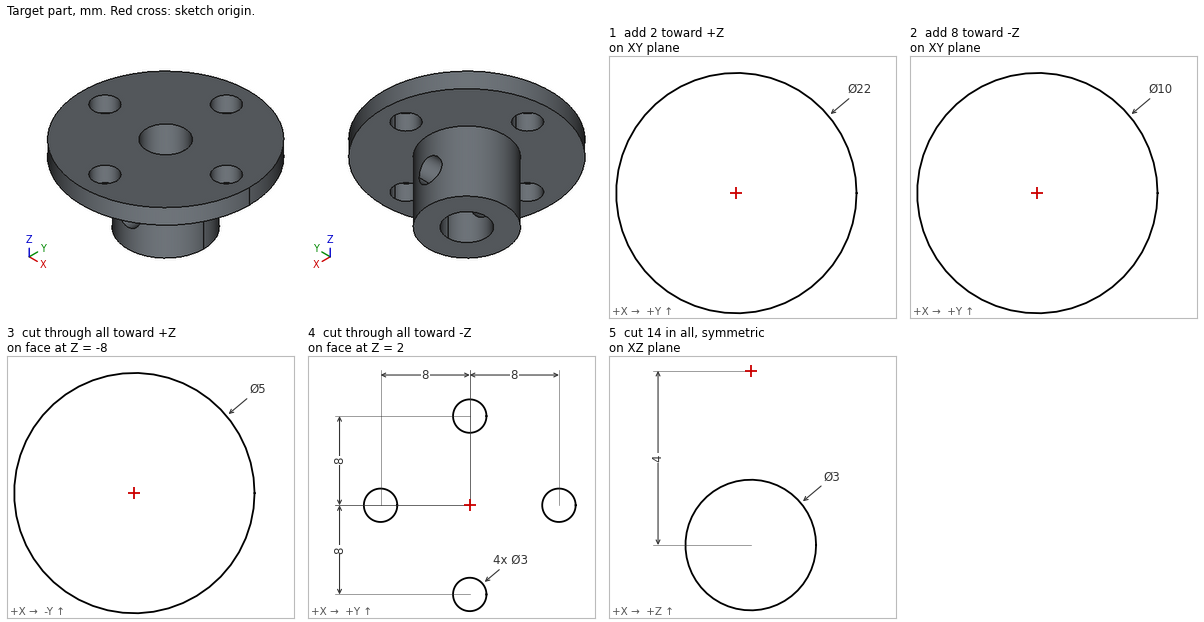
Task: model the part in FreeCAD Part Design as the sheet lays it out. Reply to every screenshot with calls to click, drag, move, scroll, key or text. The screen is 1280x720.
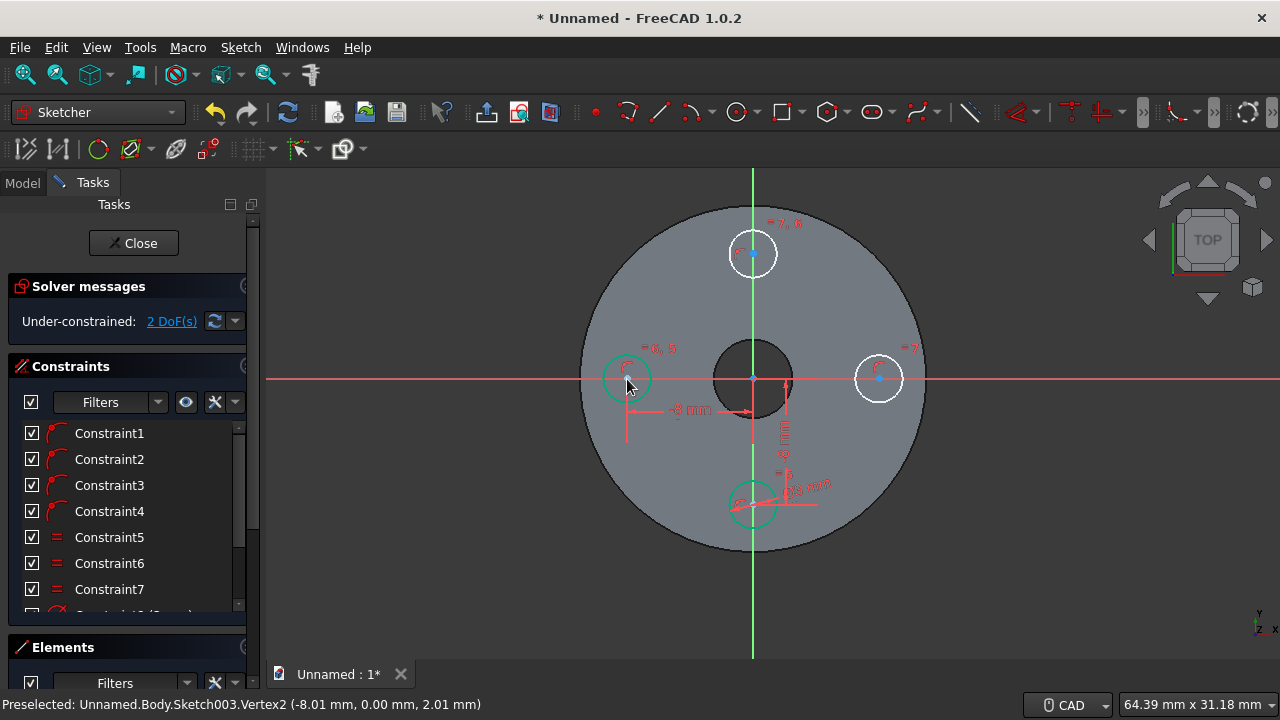
click(753, 254)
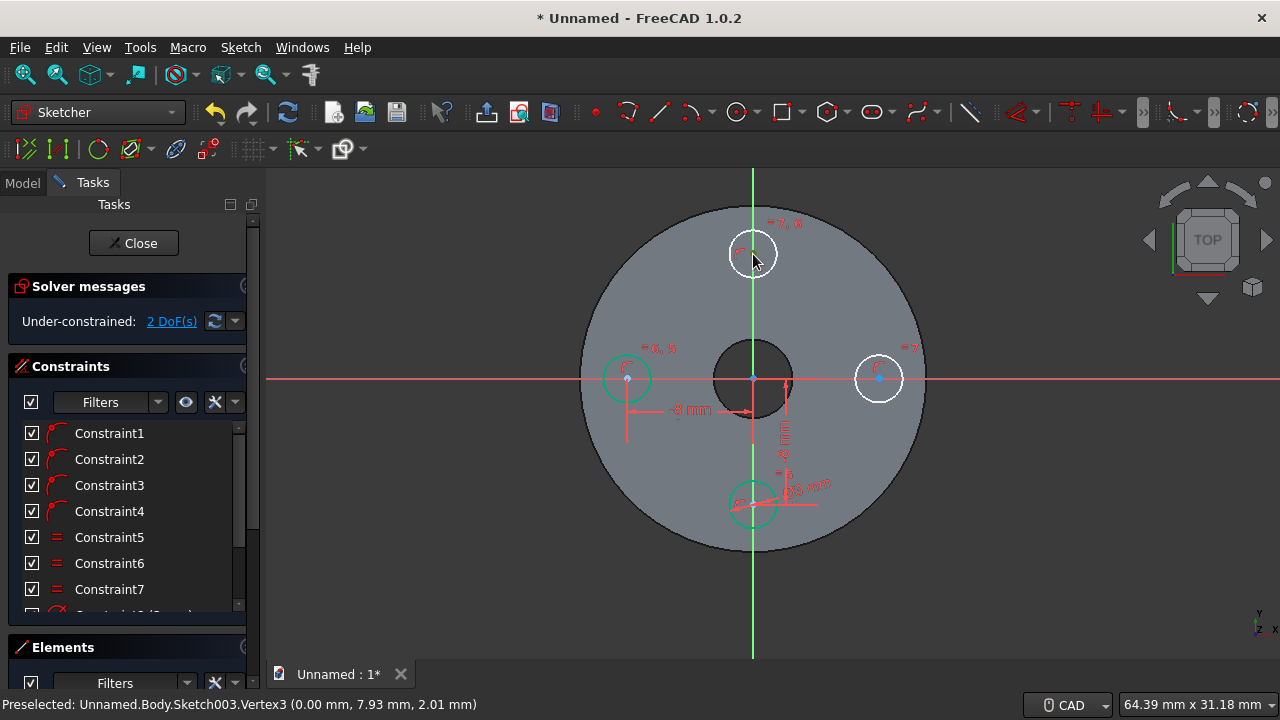
key(i)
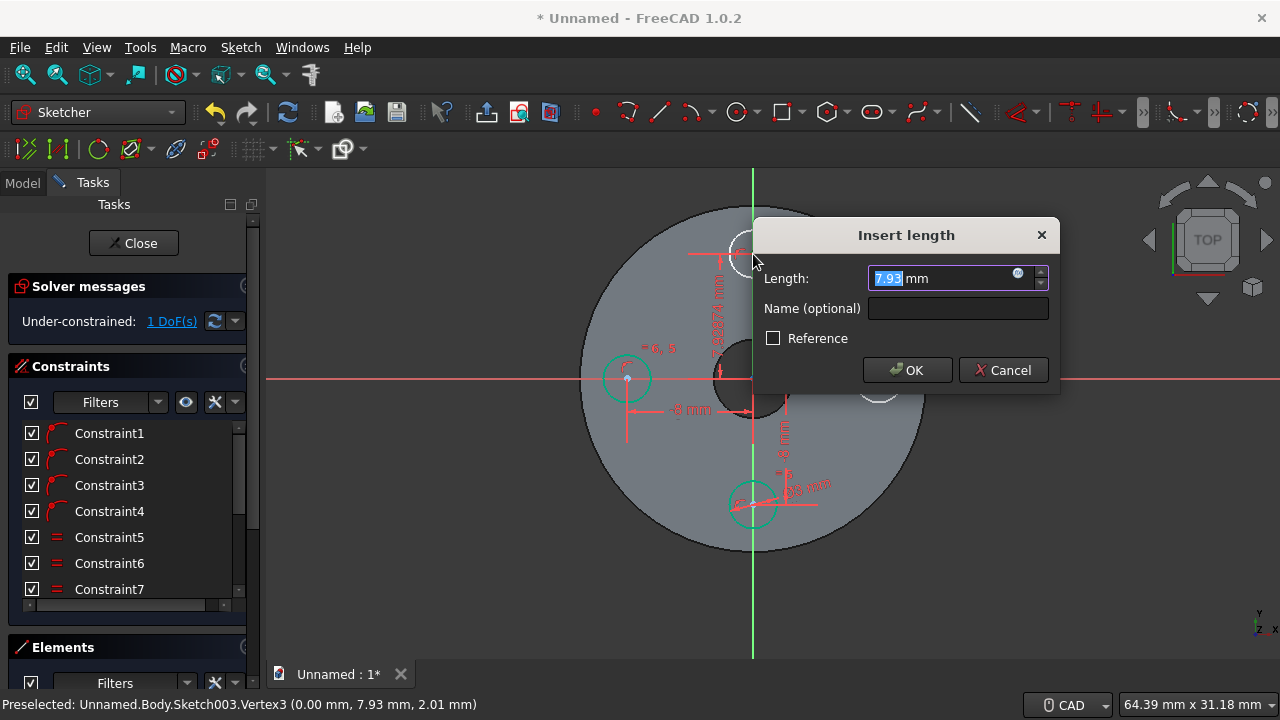
text(8)
key(Return)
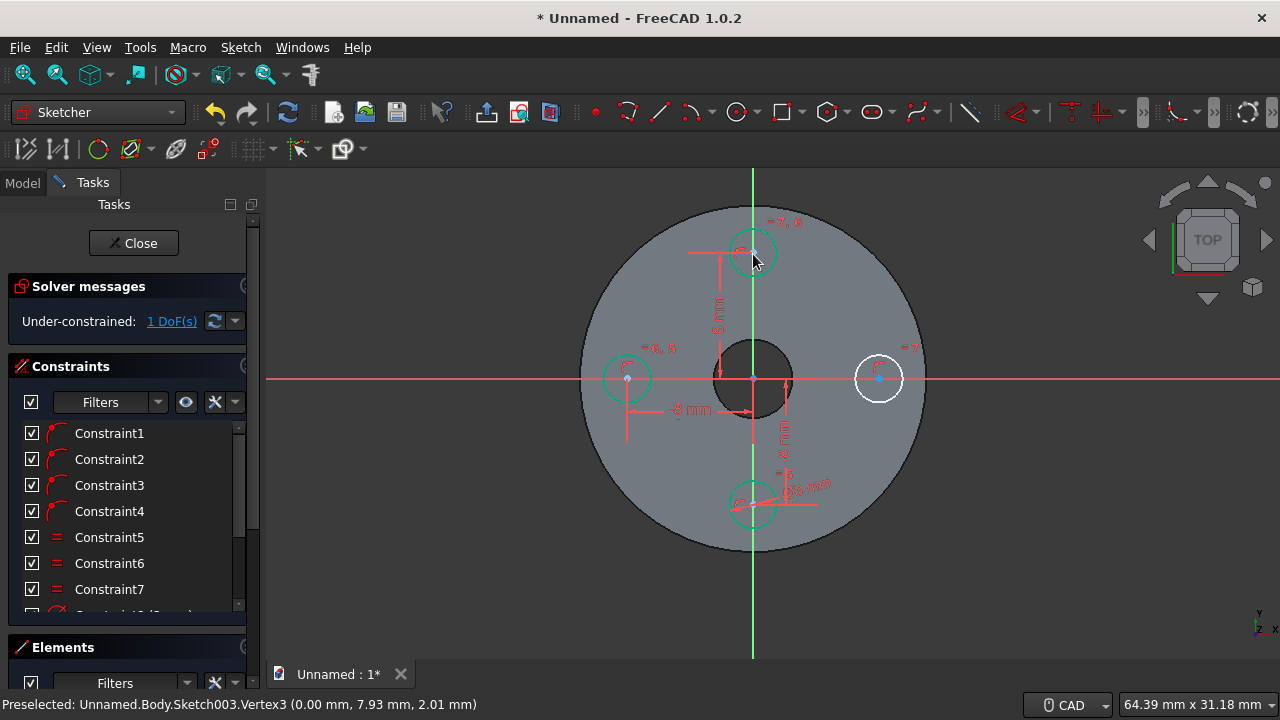
click(879, 379)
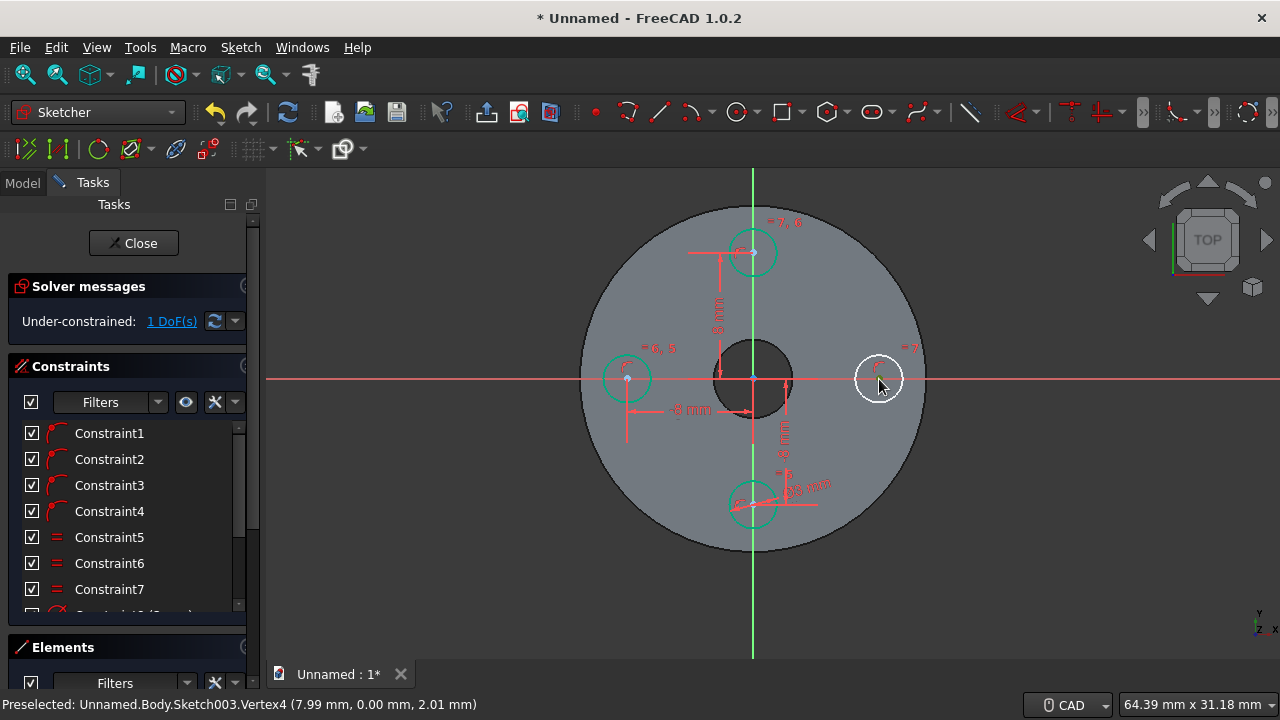
key(l)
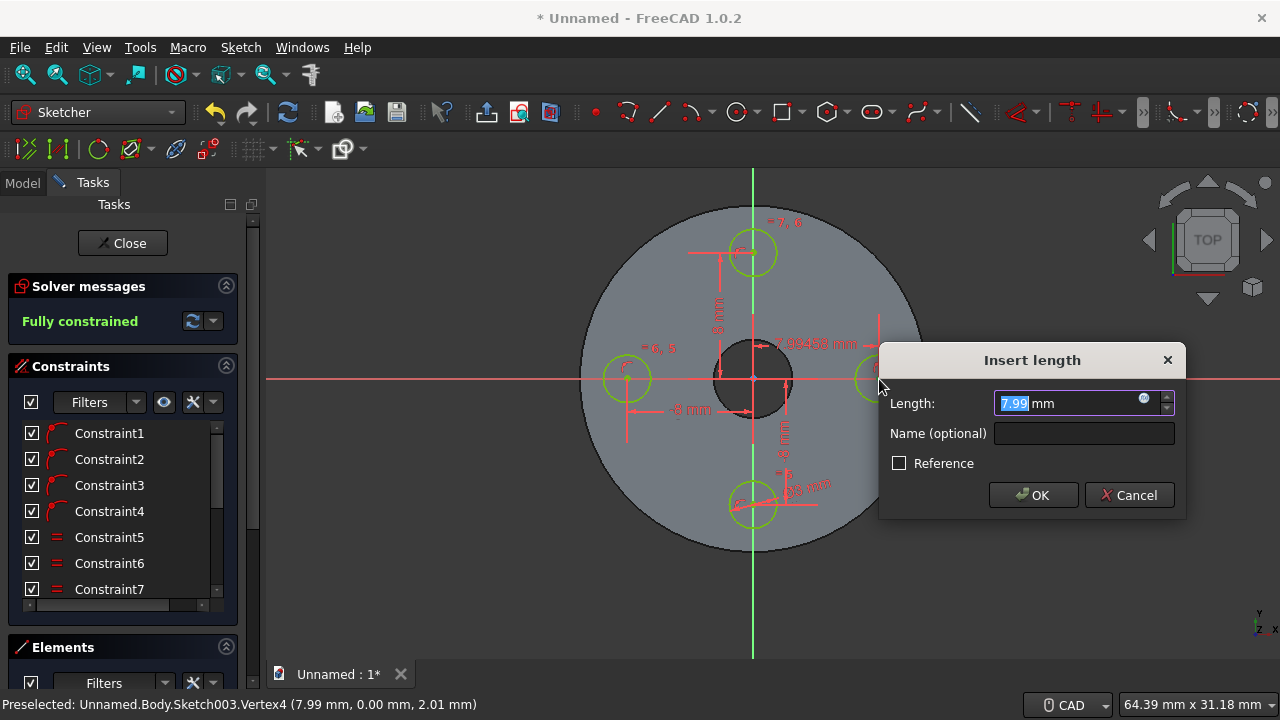
text(8)
key(Return)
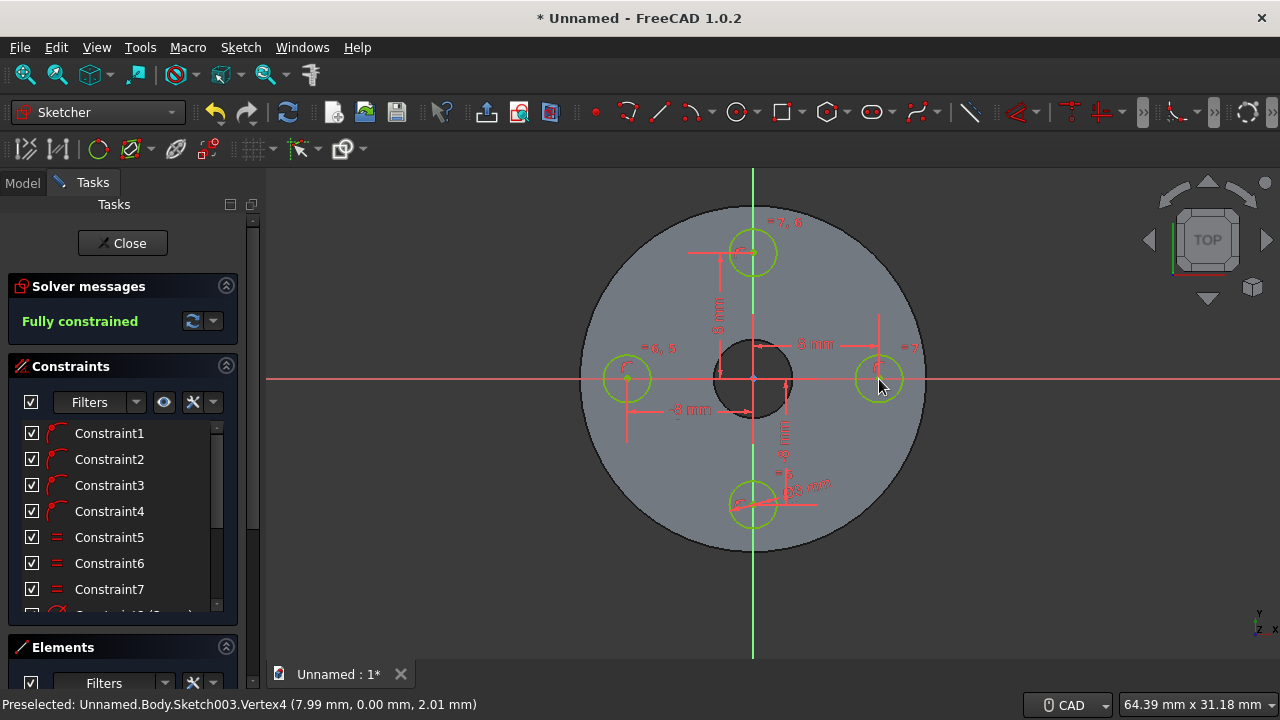
click(123, 243)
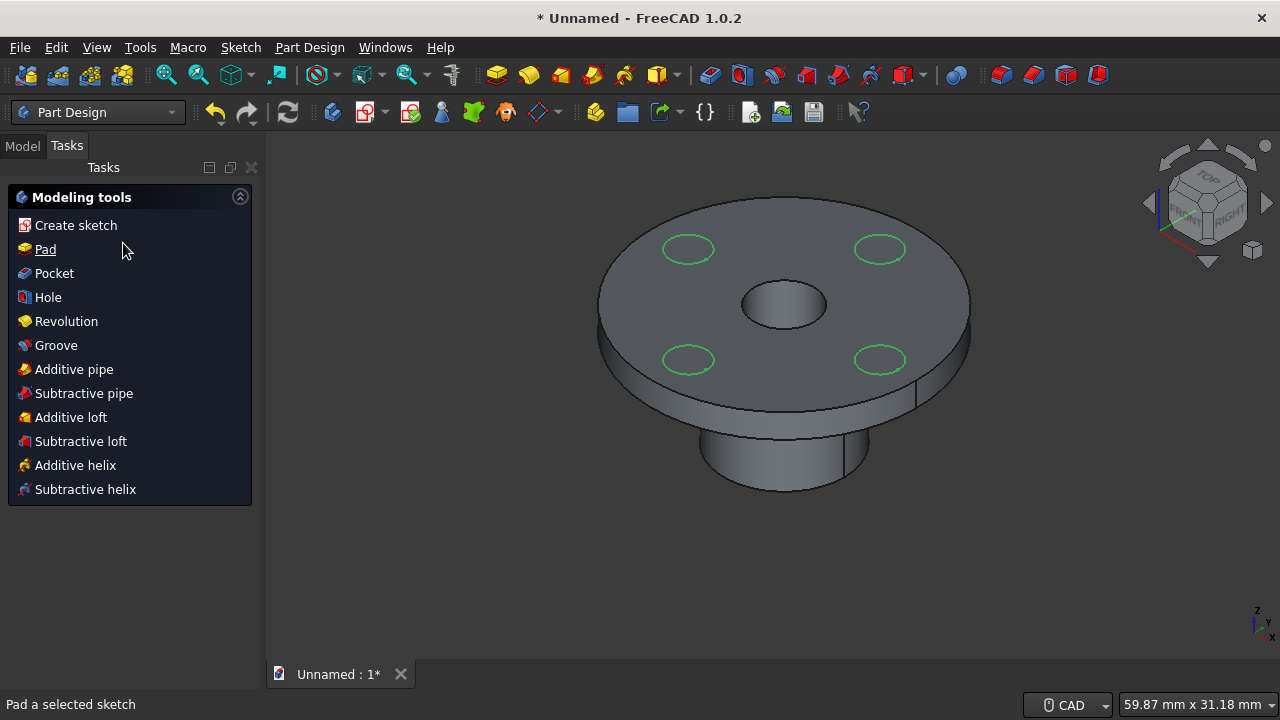
click(712, 76)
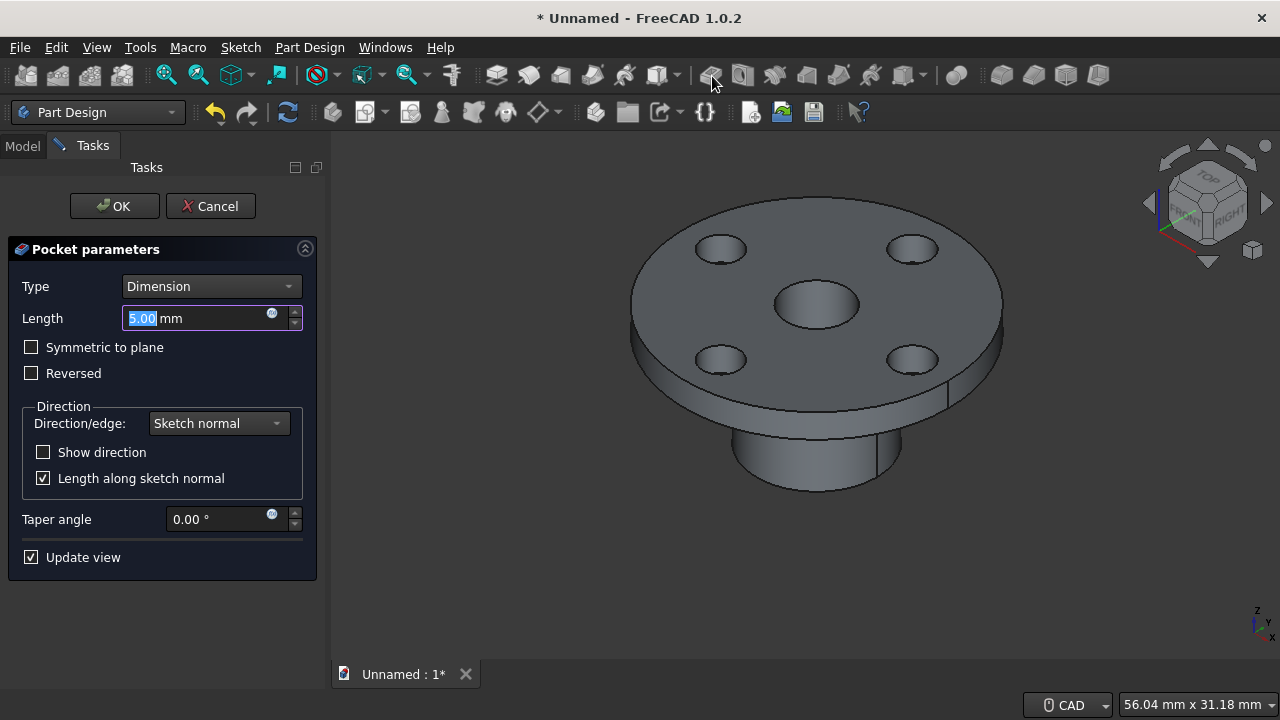
click(212, 286)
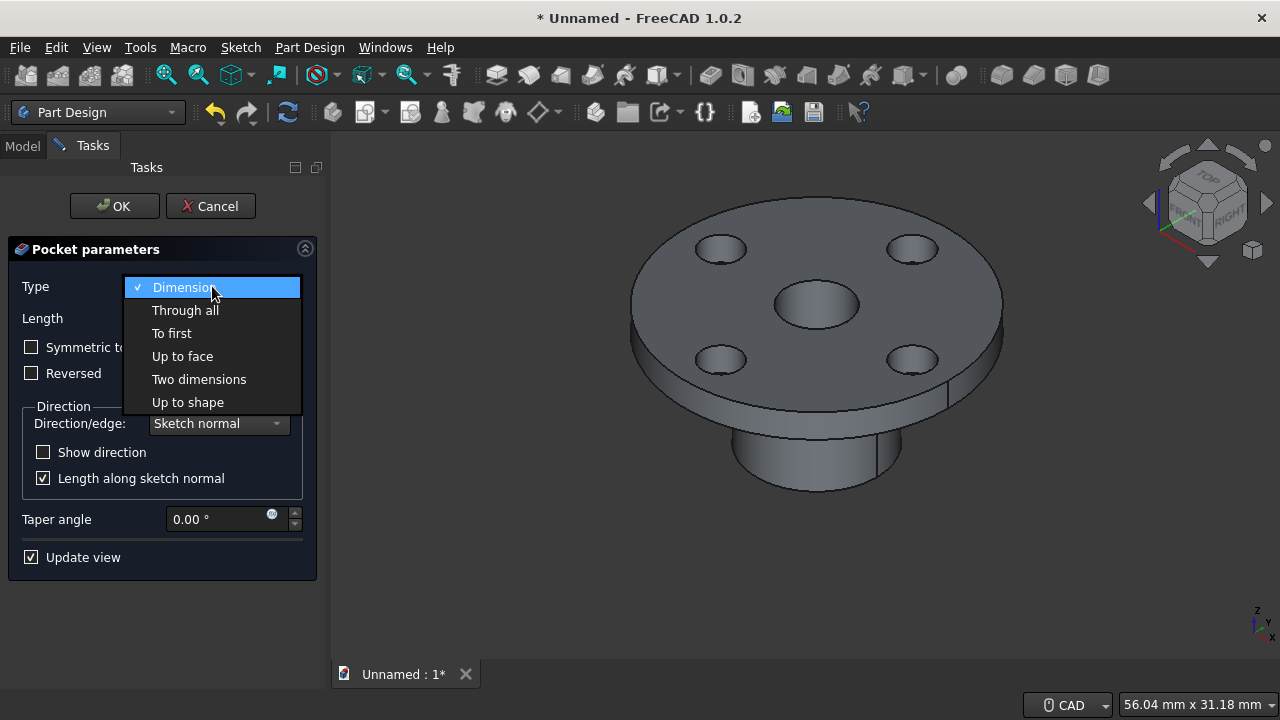
click(212, 310)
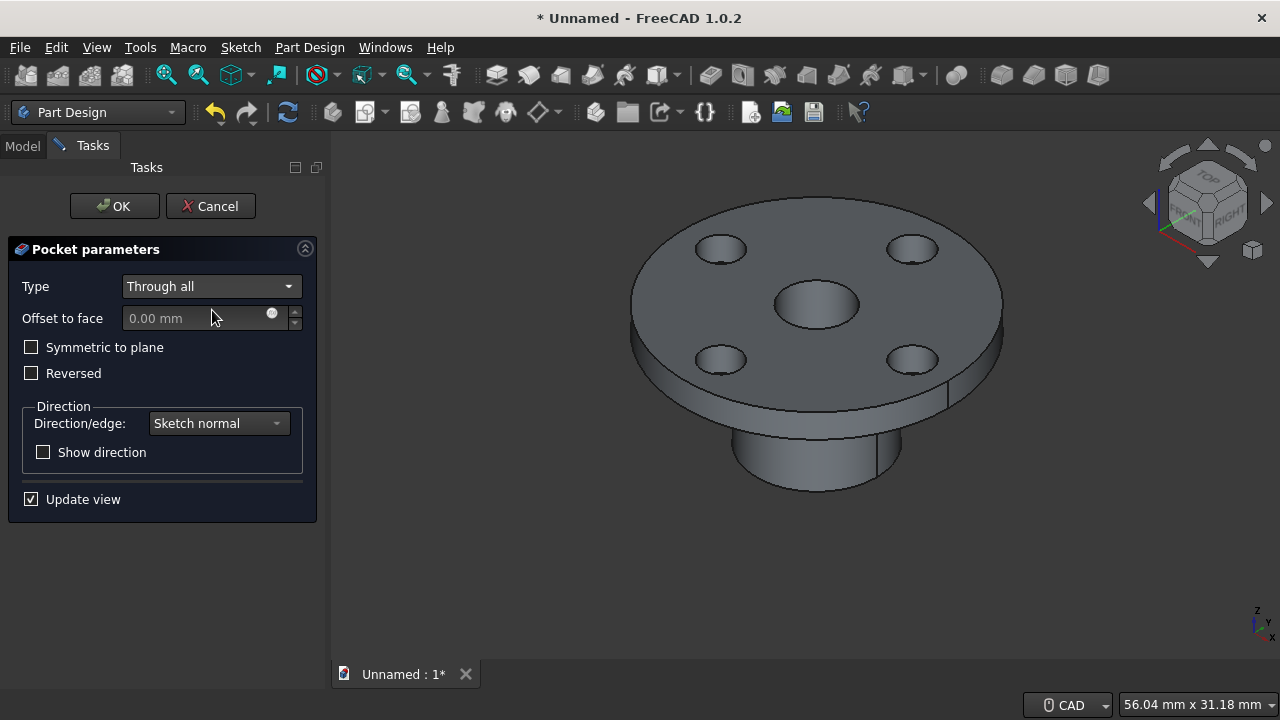
click(115, 206)